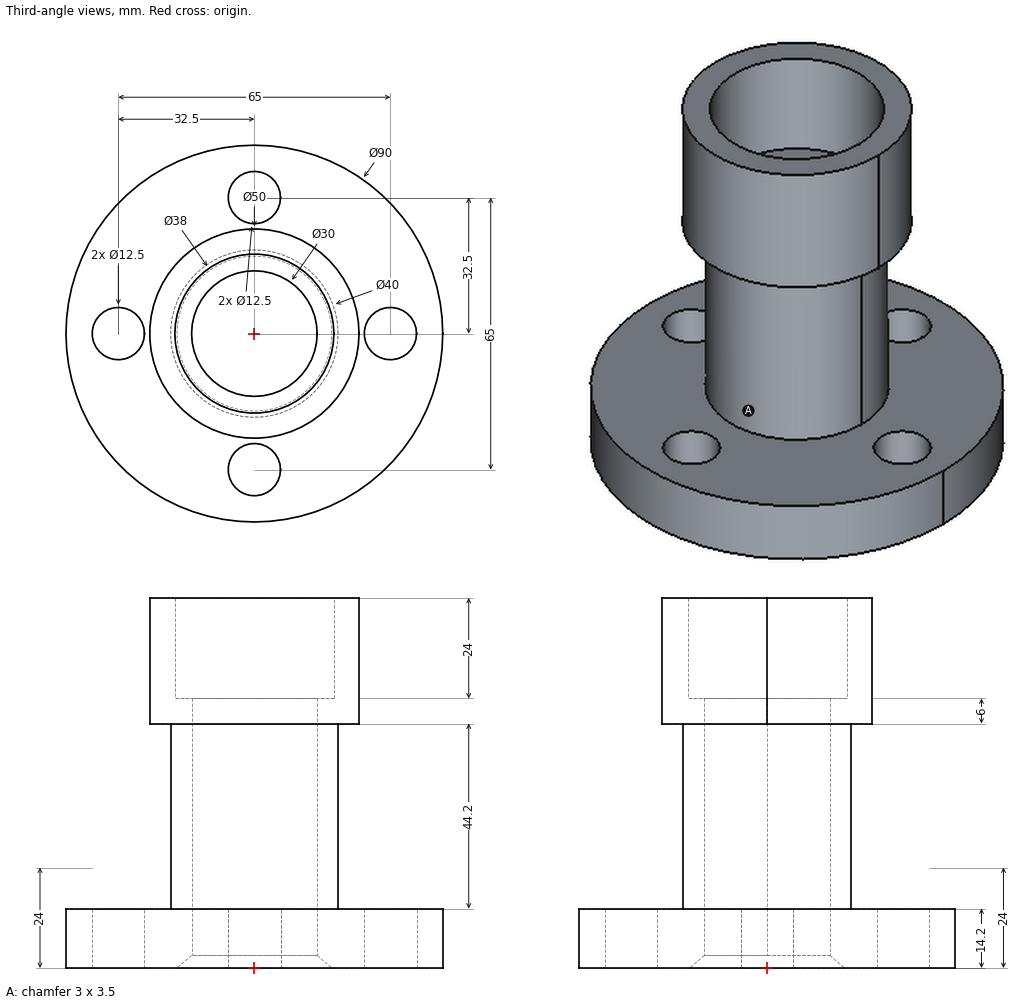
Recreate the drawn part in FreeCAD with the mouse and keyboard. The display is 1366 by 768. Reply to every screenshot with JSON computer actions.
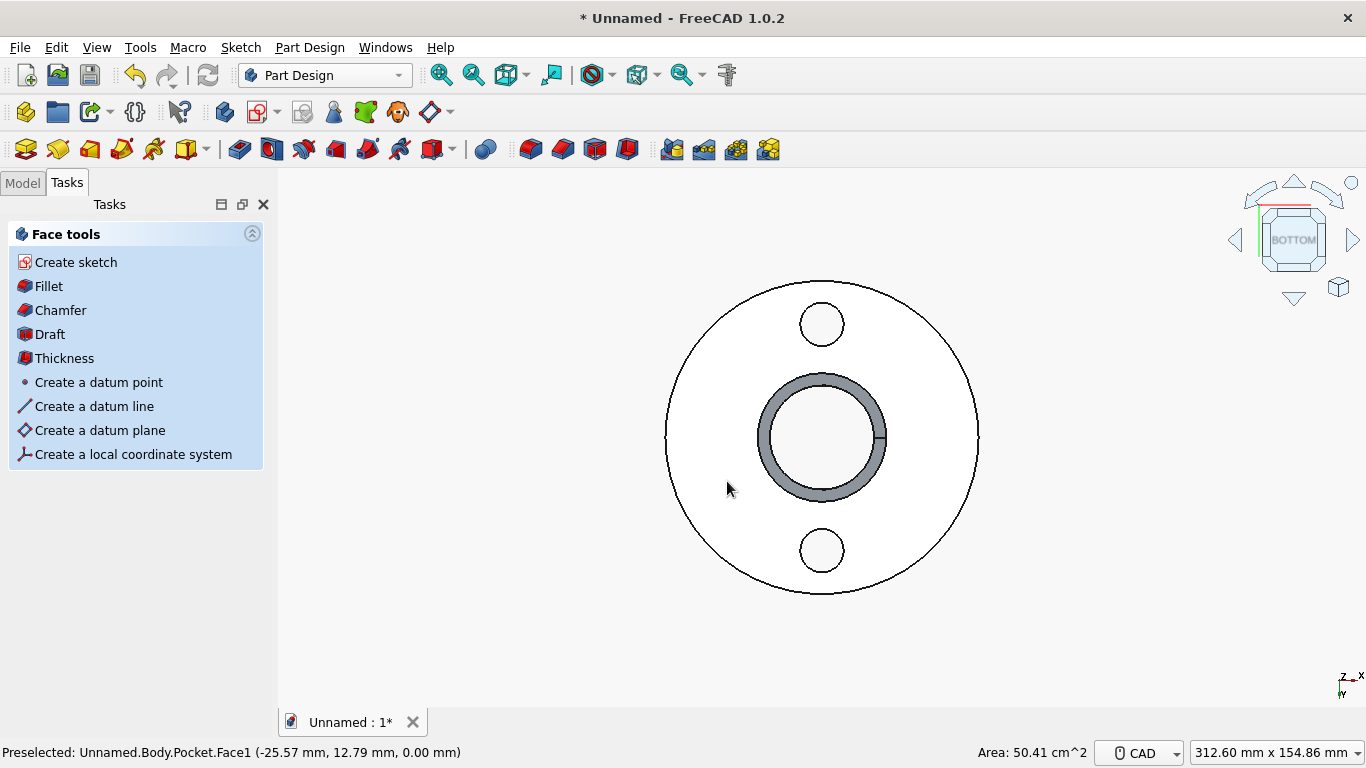
{"action": "left_click", "coordinate": [258, 112]}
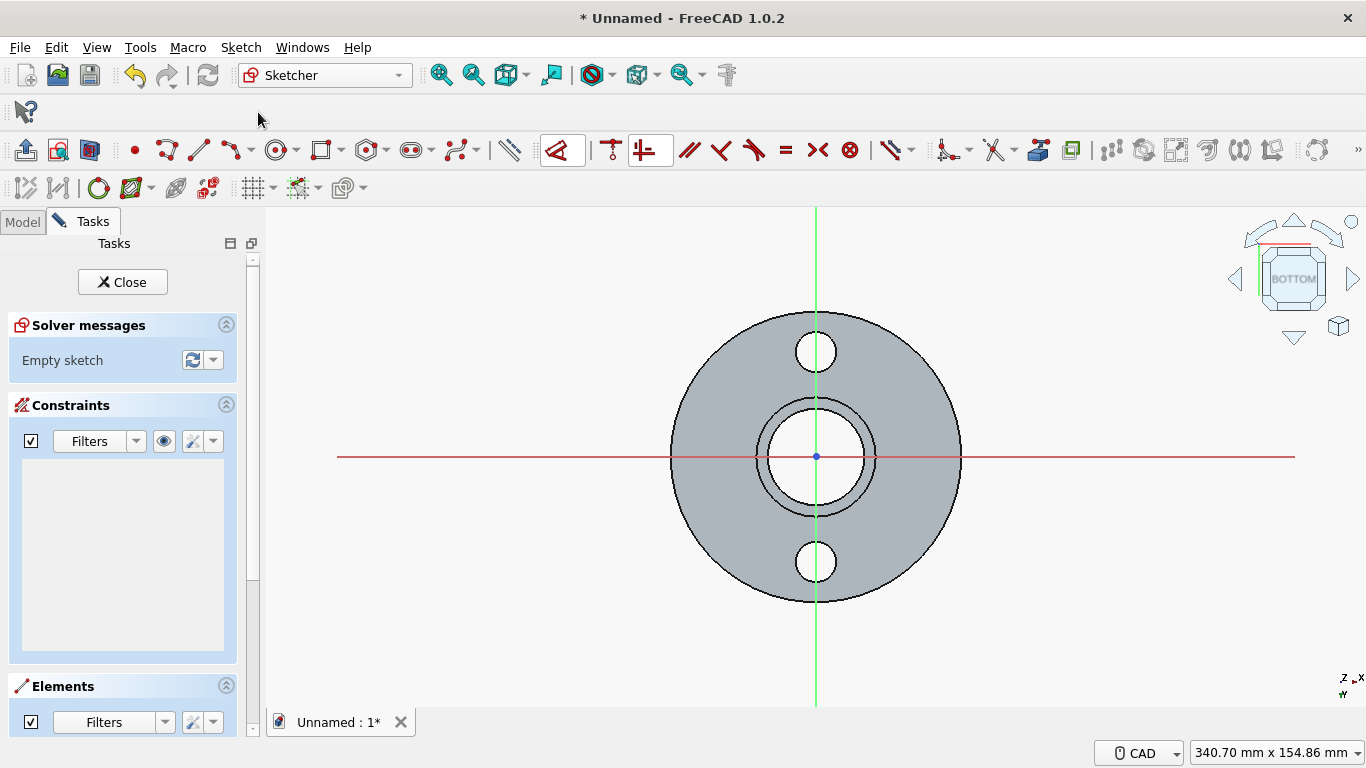
{"action": "scroll", "coordinate": [856, 457], "scroll_direction": "up", "scroll_amount": 5}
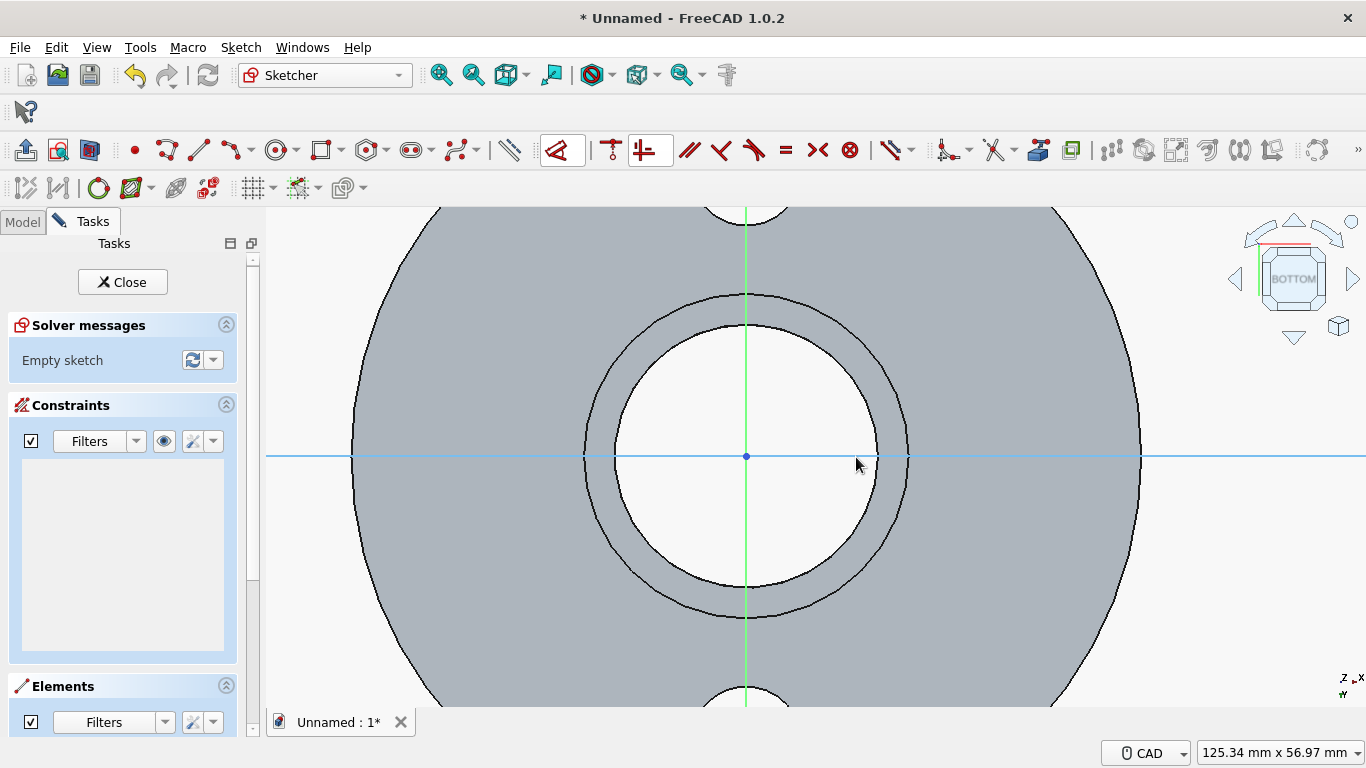
{"action": "key", "text": "g c"}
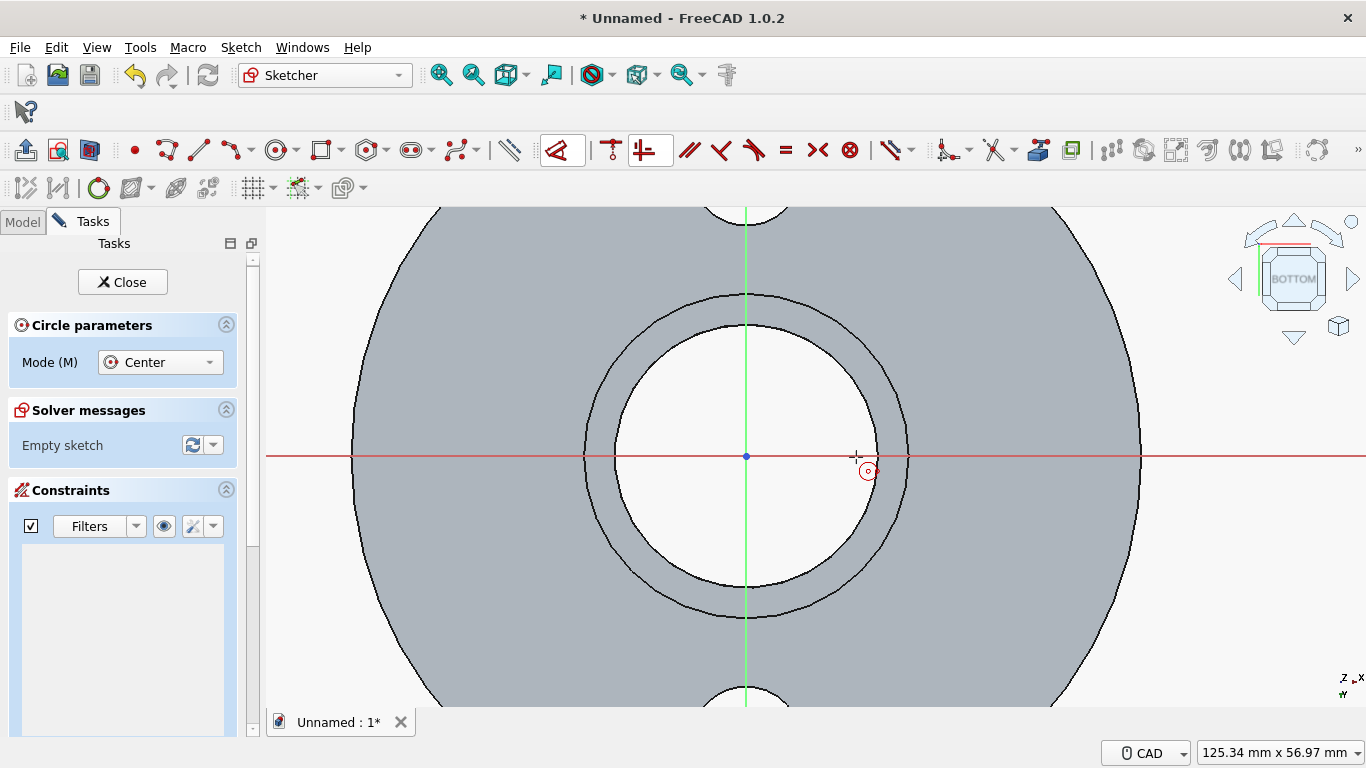
{"action": "left_click", "coordinate": [461, 456]}
{"action": "mouse_move", "coordinate": [500, 417]}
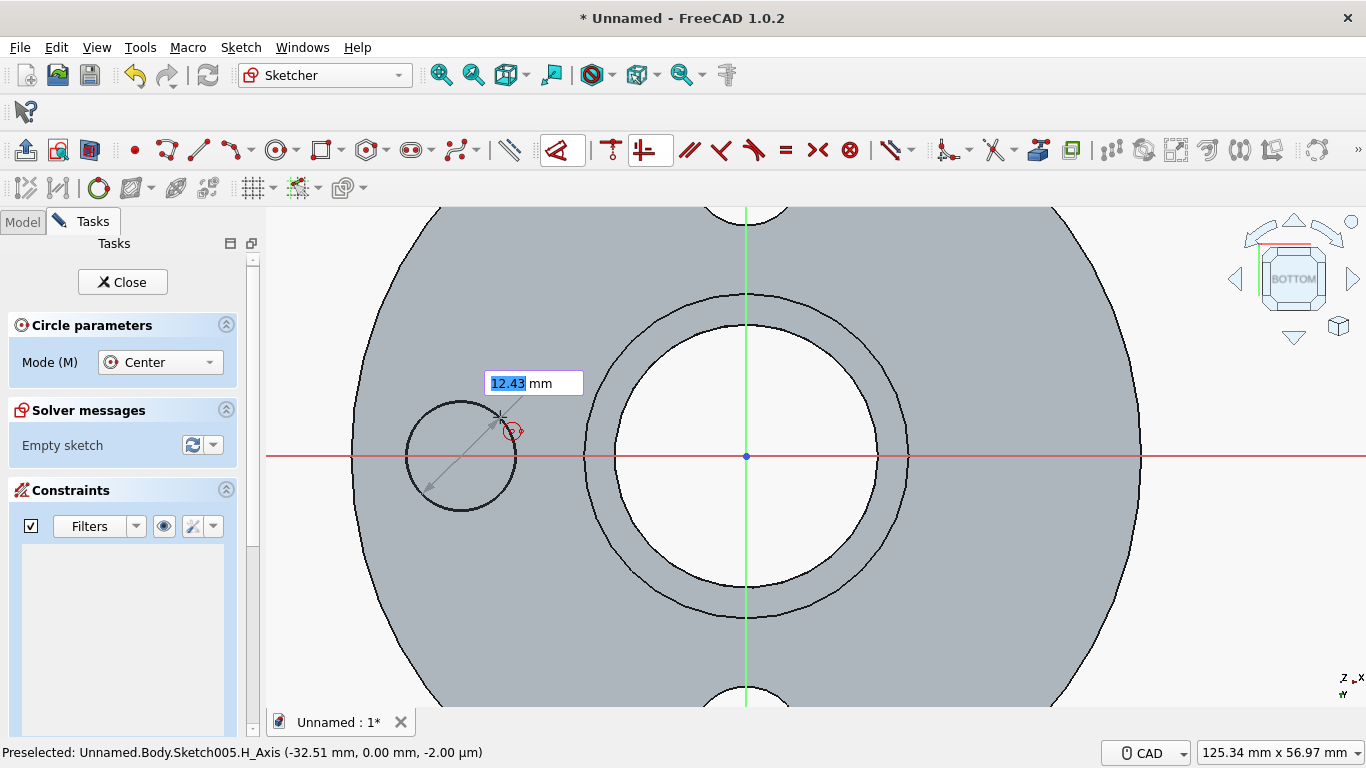
{"action": "type", "text": "12.5"}
{"action": "key", "text": "Return"}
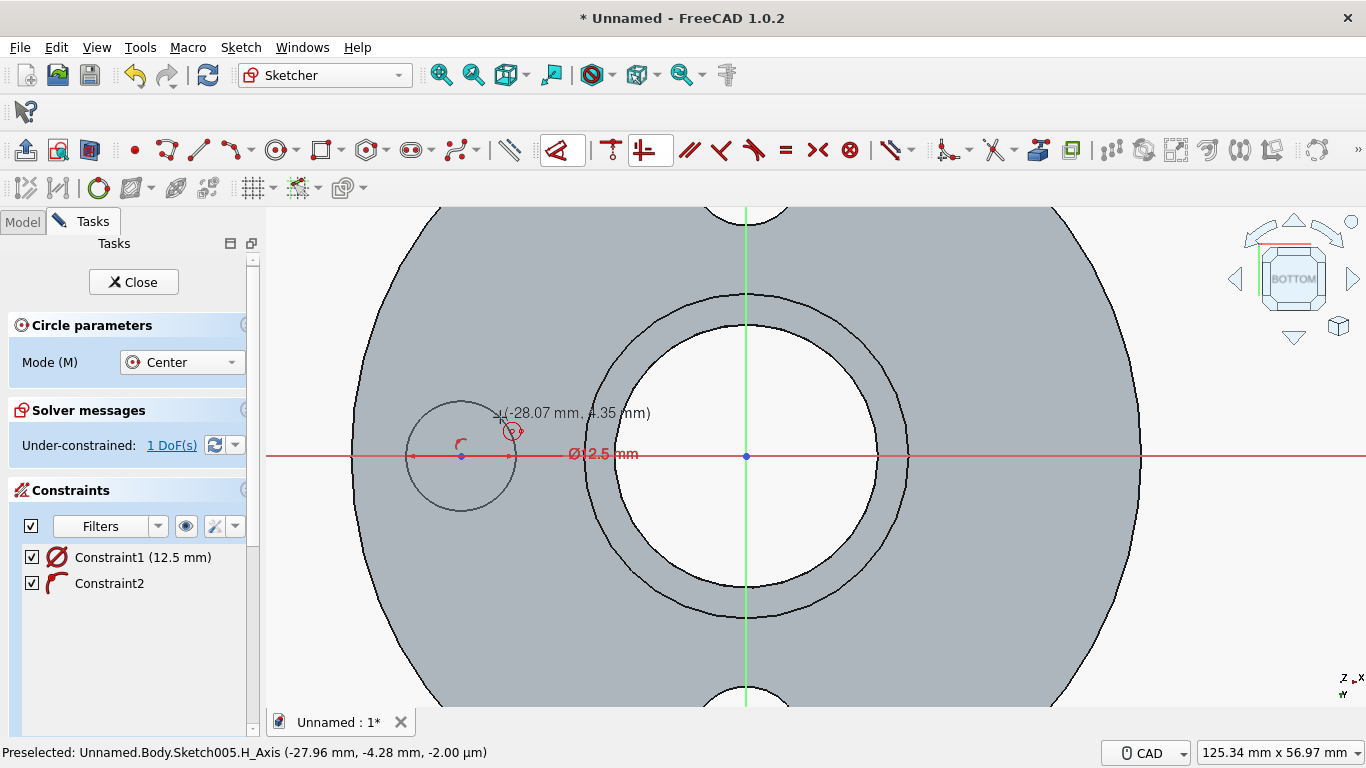
{"action": "left_click", "coordinate": [1032, 456]}
{"action": "mouse_move", "coordinate": [1070, 417]}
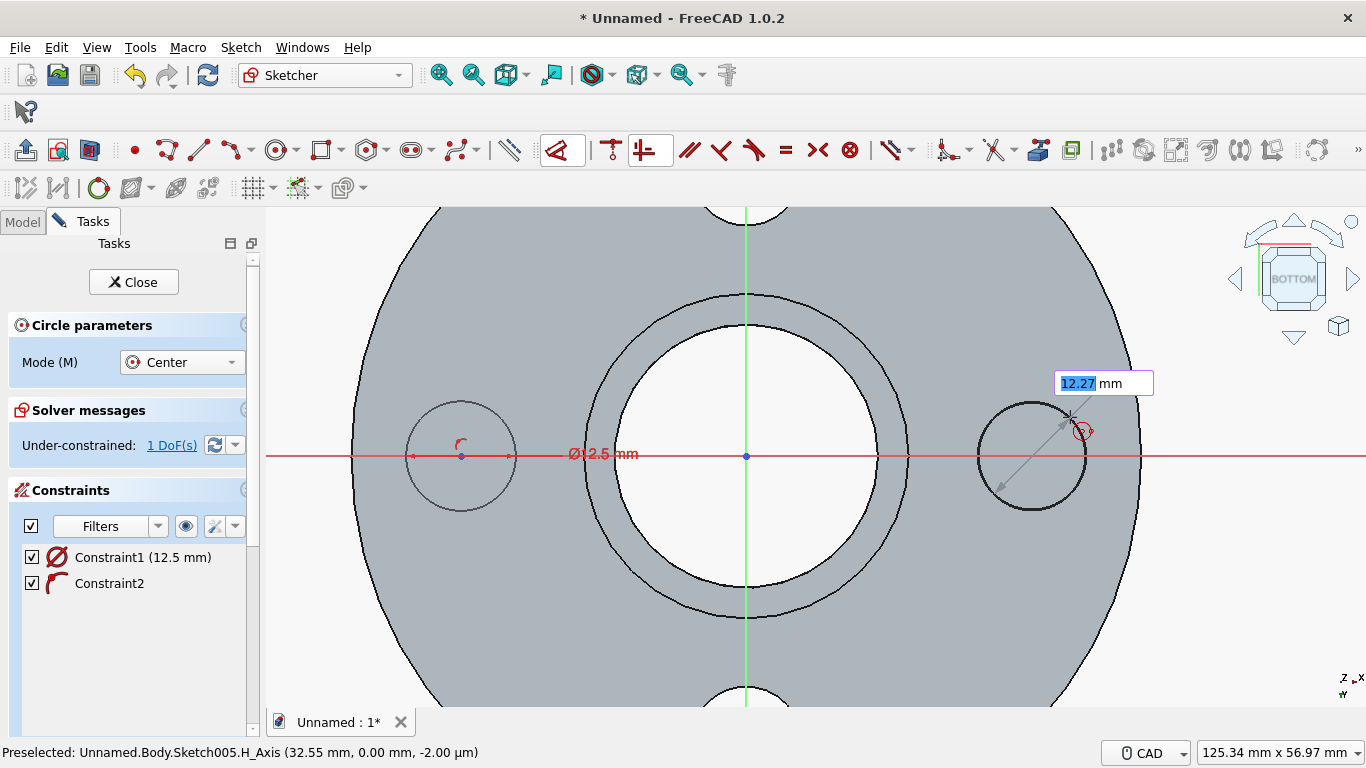
{"action": "type", "text": "12.5"}
{"action": "key", "text": "Return"}
{"action": "key", "text": "Escape"}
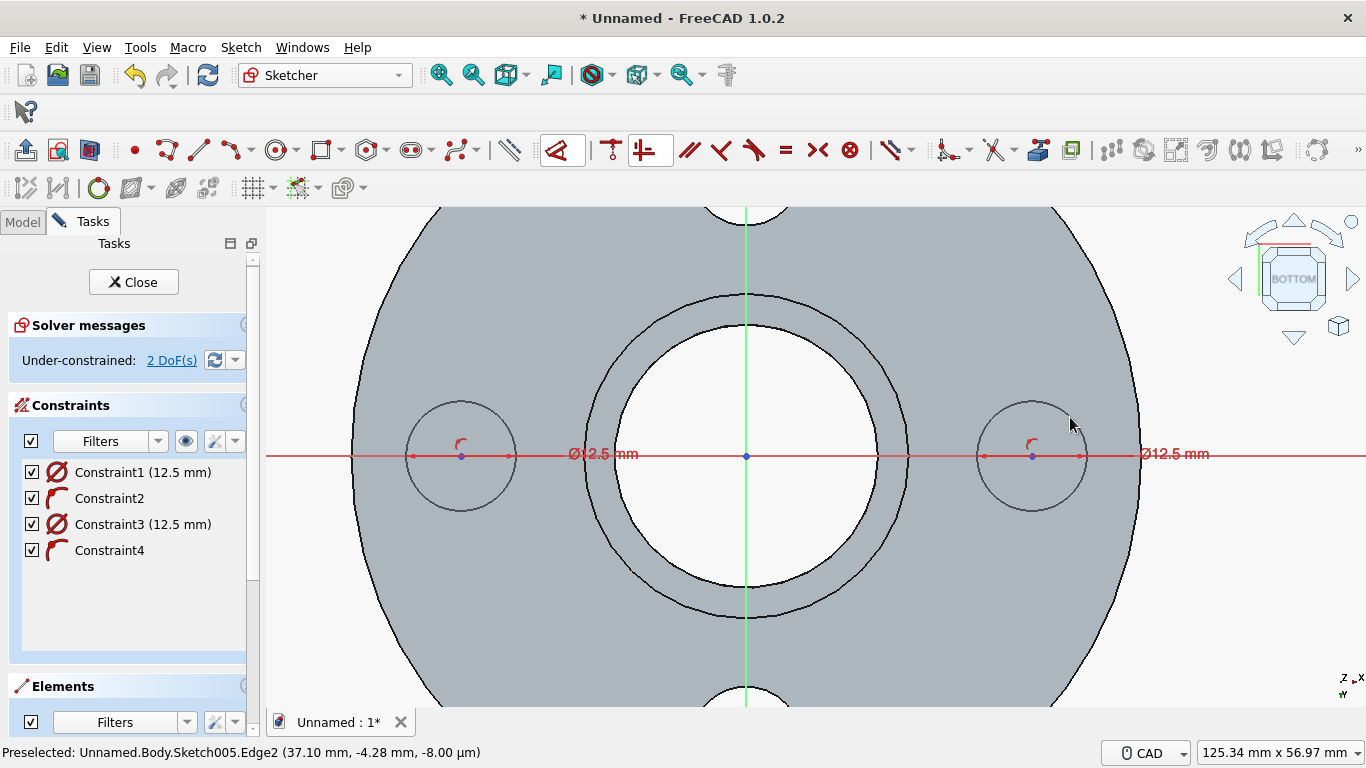
{"action": "left_click", "coordinate": [461, 456]}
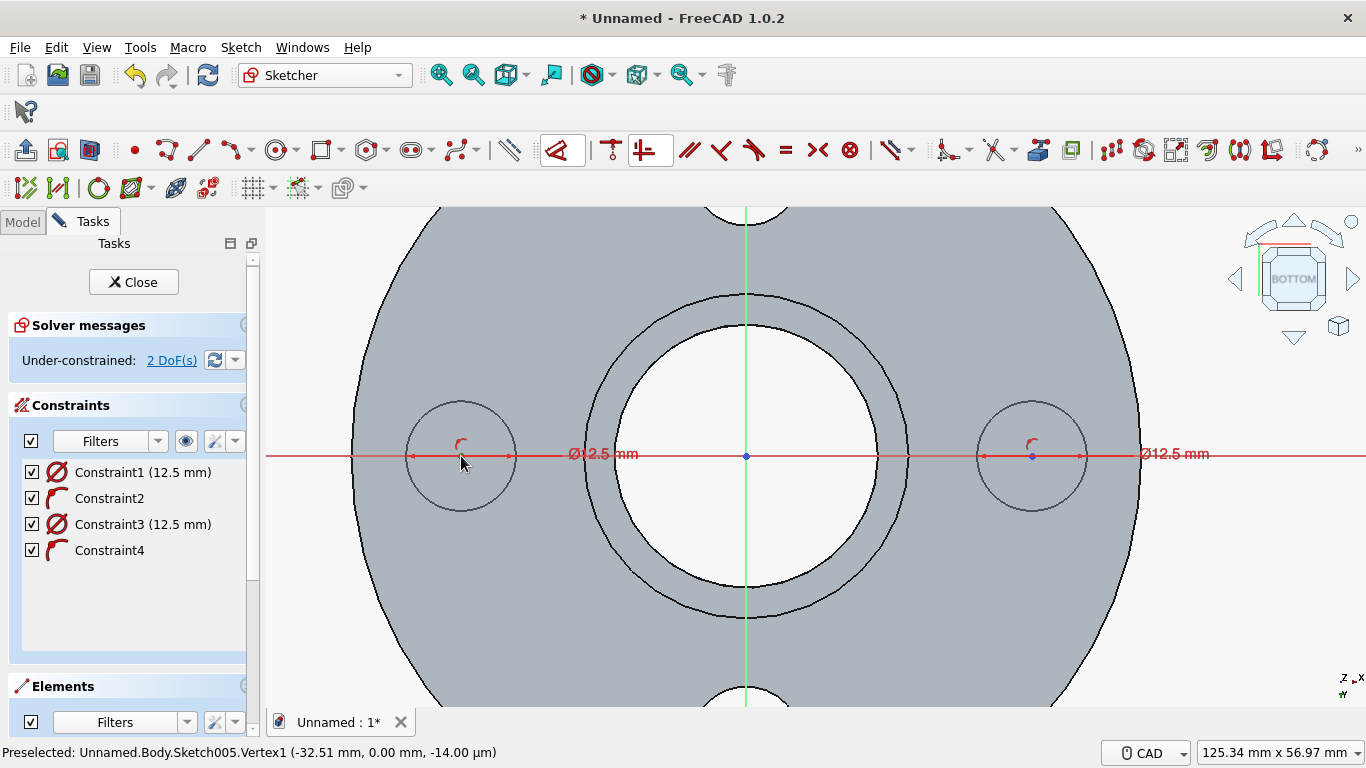
{"action": "left_click", "coordinate": [1032, 456]}